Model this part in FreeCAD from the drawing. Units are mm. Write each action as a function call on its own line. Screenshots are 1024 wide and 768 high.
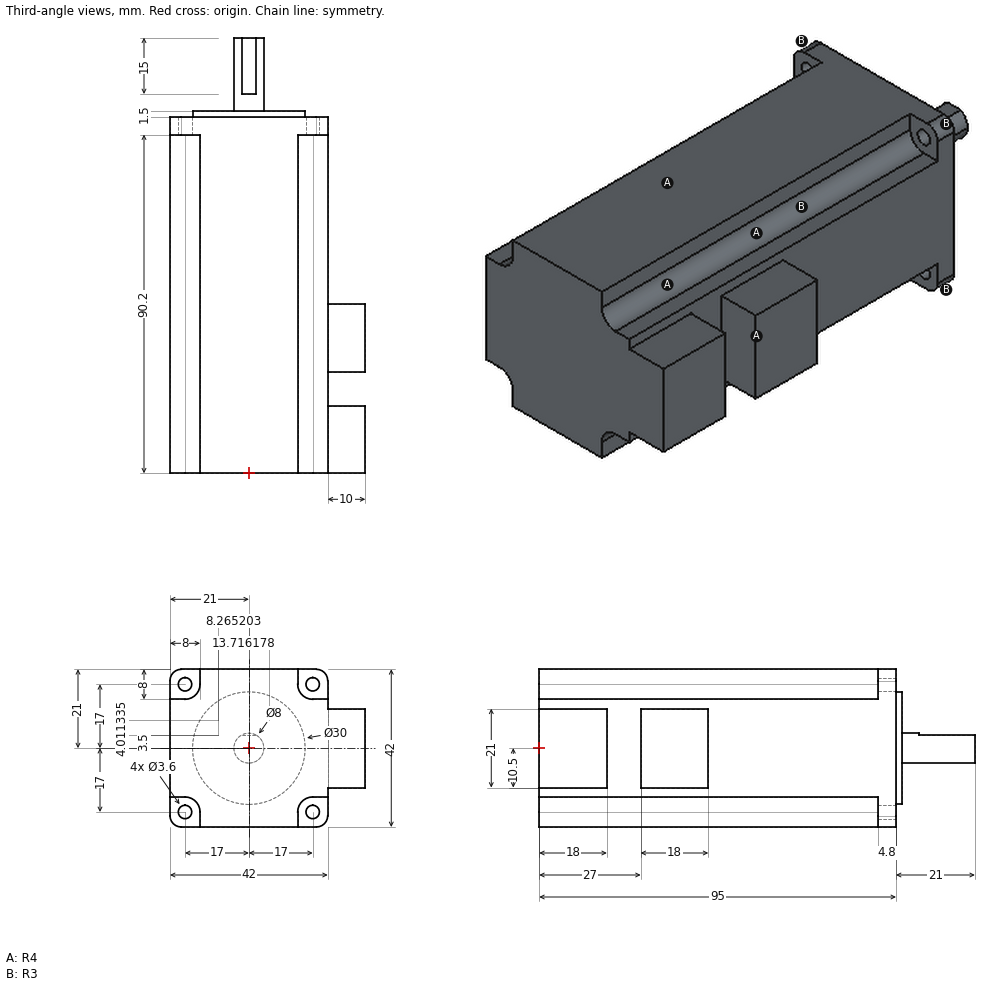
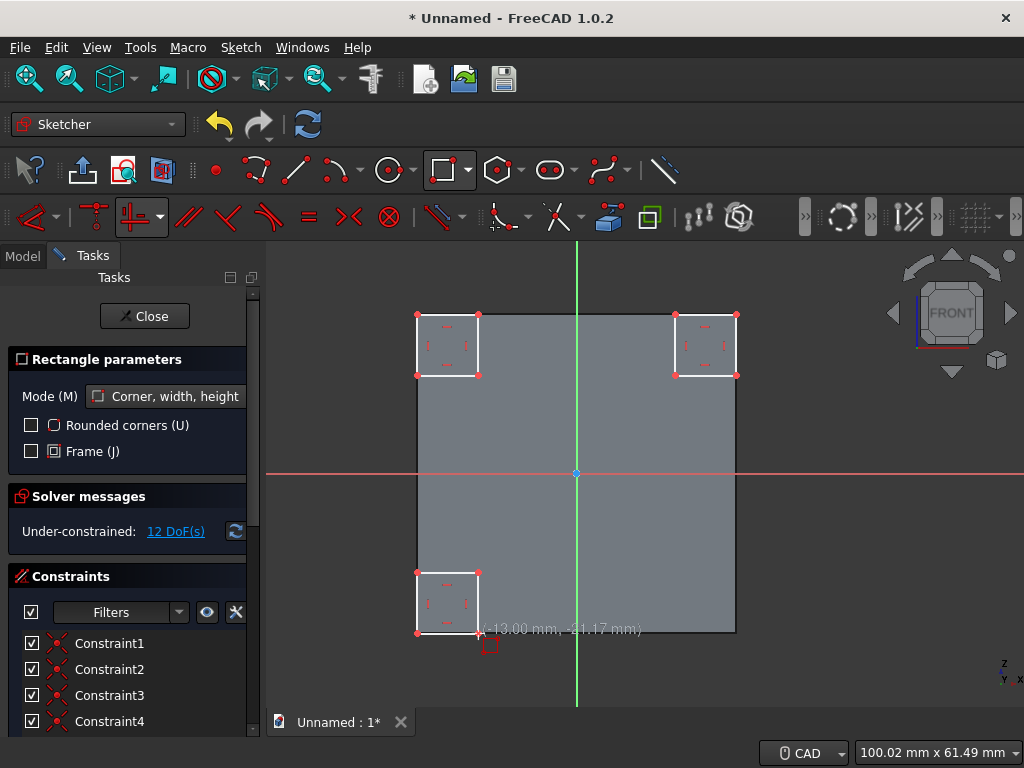
click(675, 572)
click(736, 633)
key(Escape)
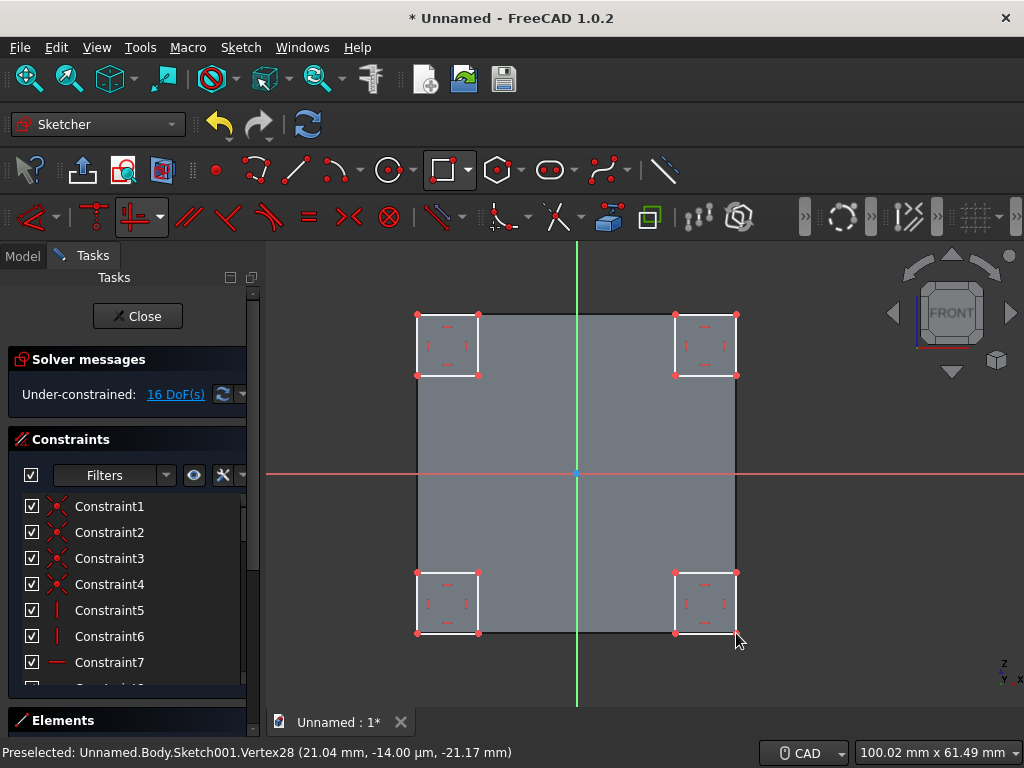
click(478, 315)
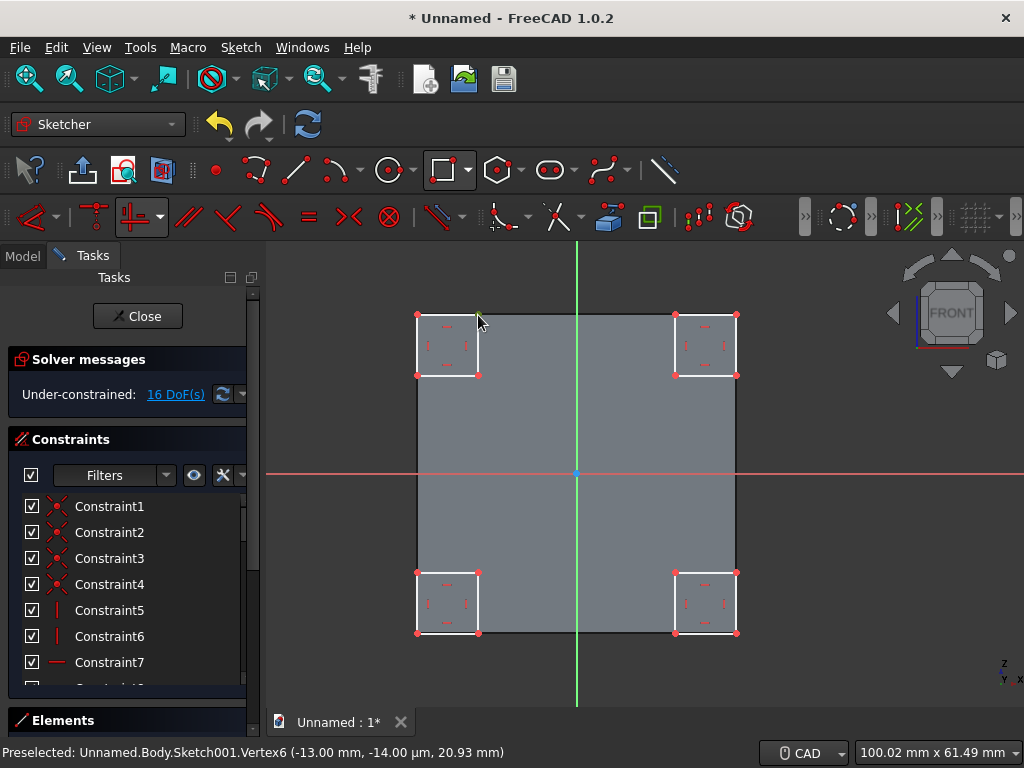
click(675, 315)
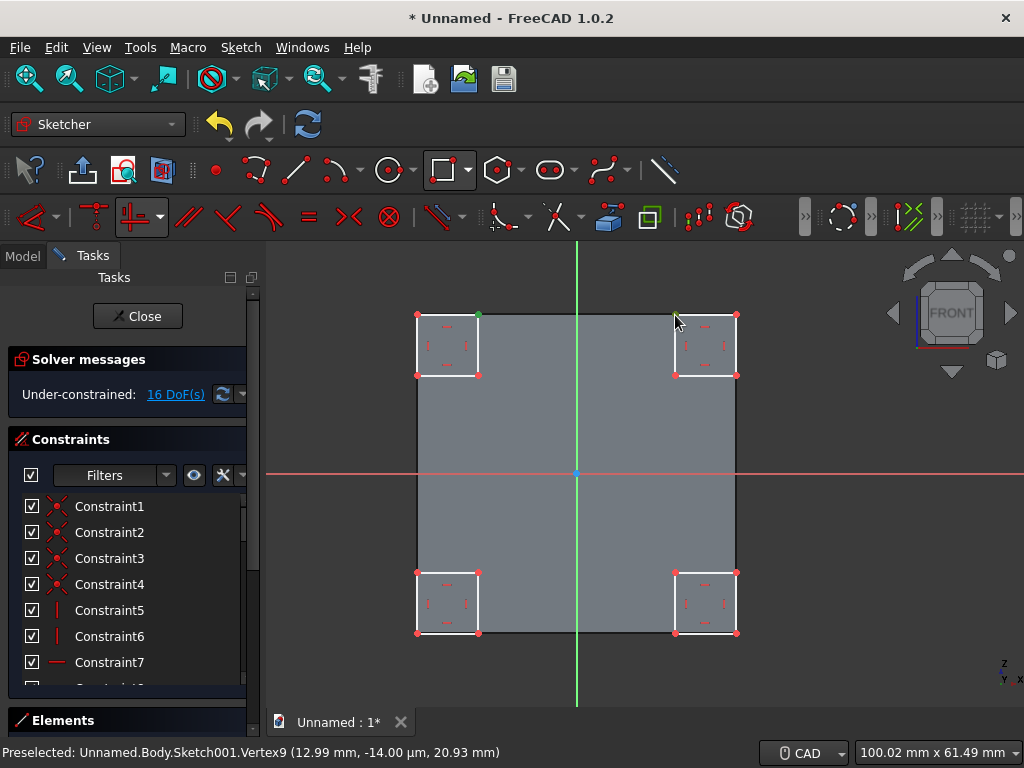
click(577, 650)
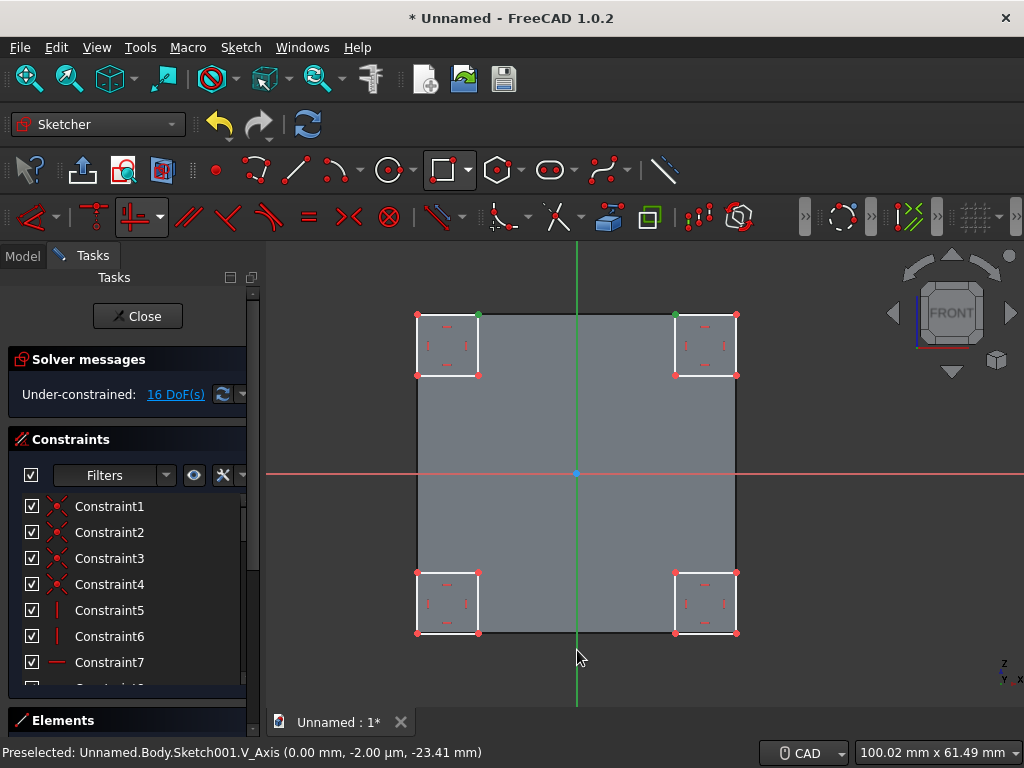
click(350, 218)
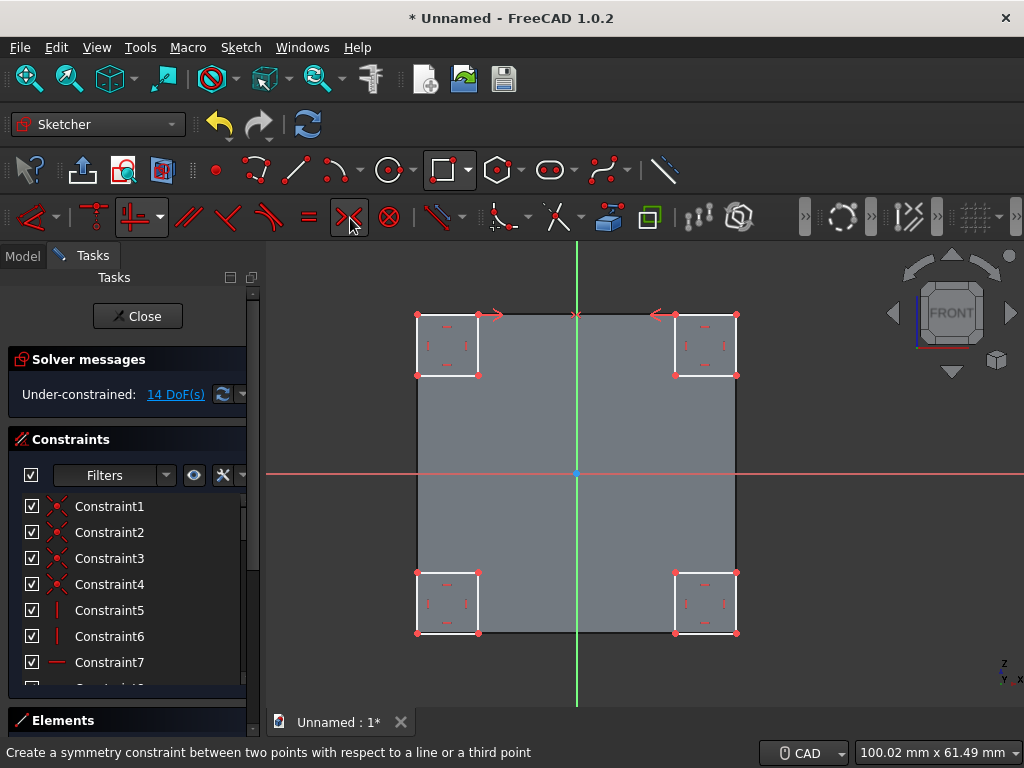
click(417, 376)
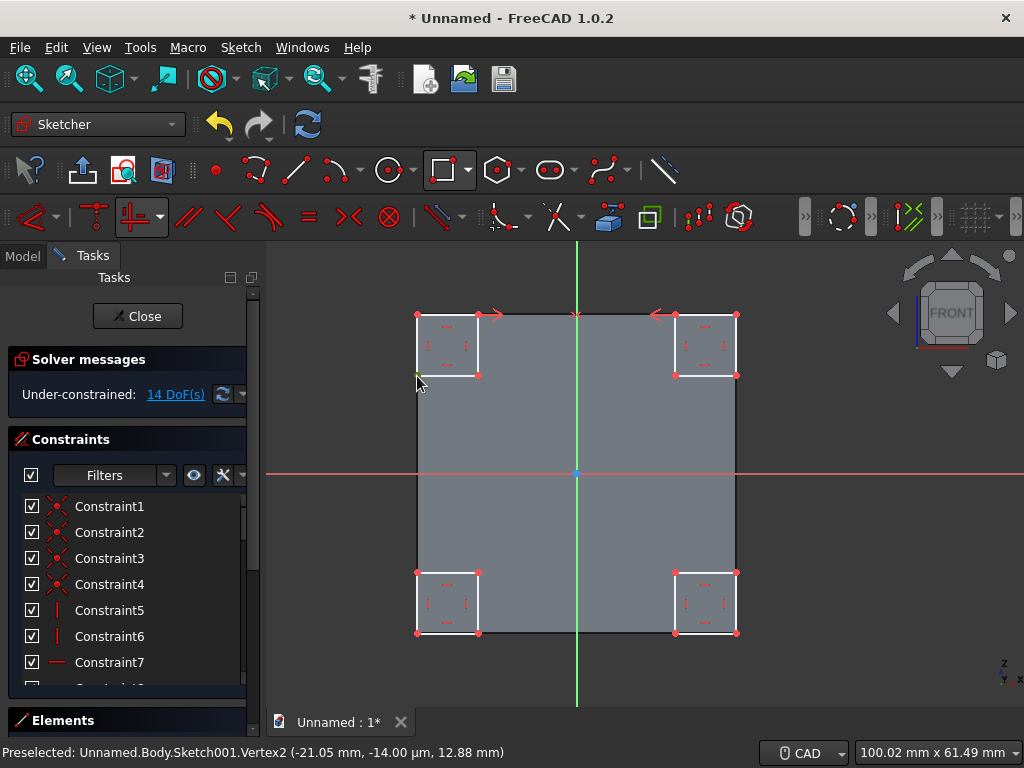
click(736, 376)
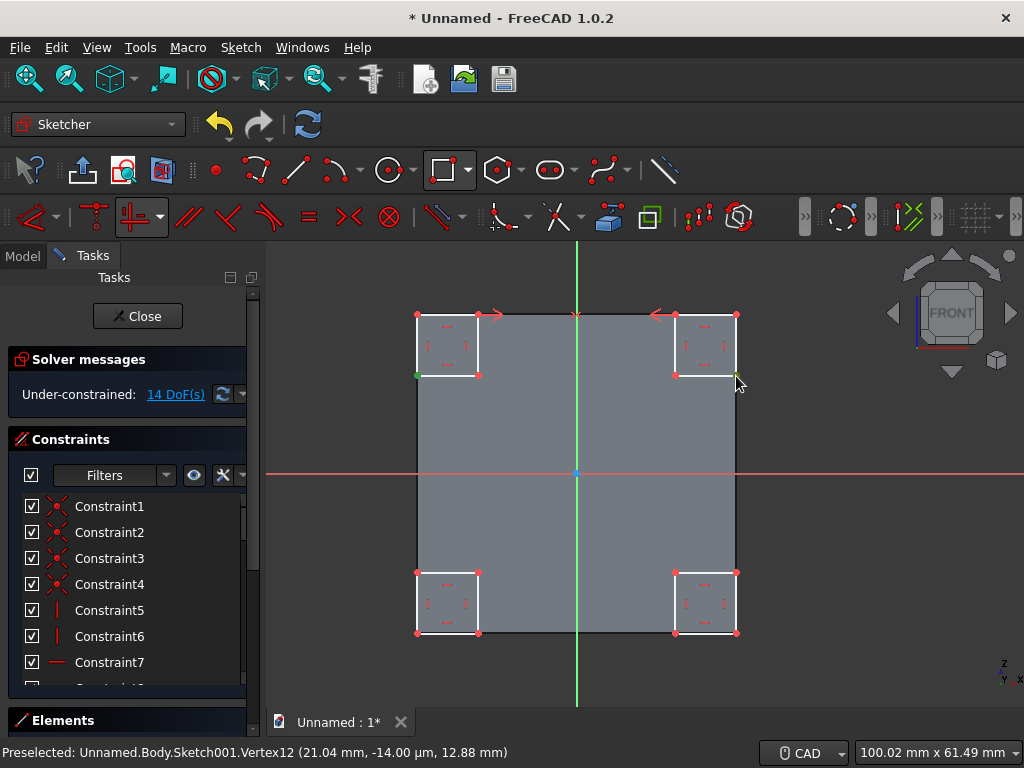
click(577, 650)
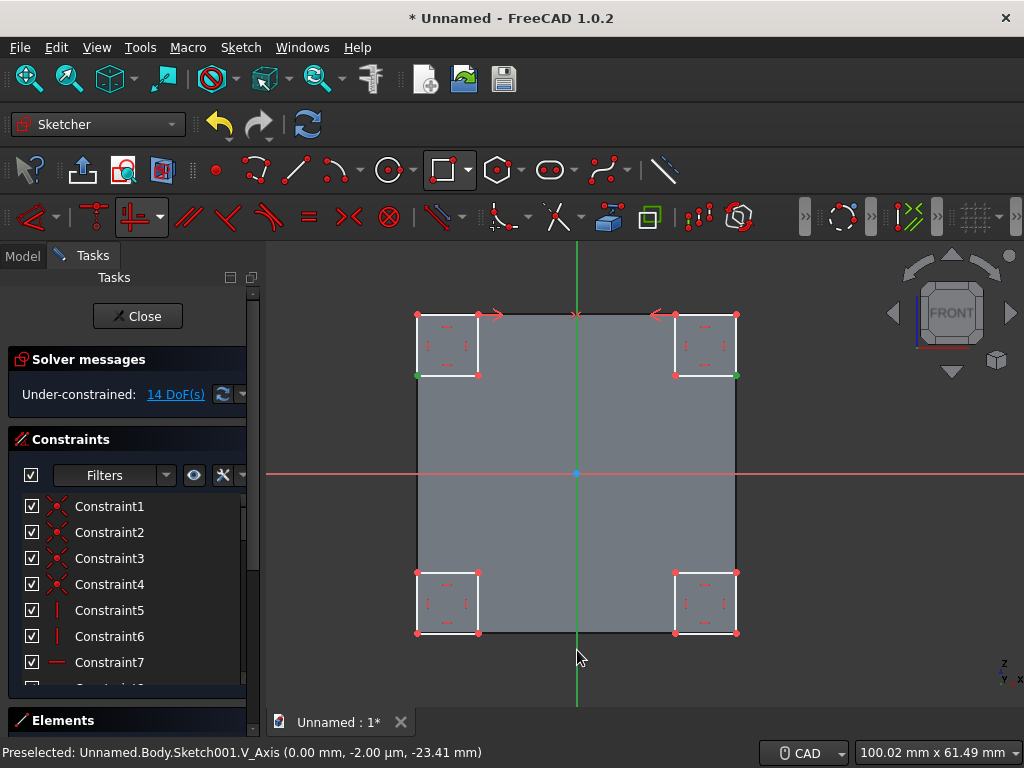
click(350, 218)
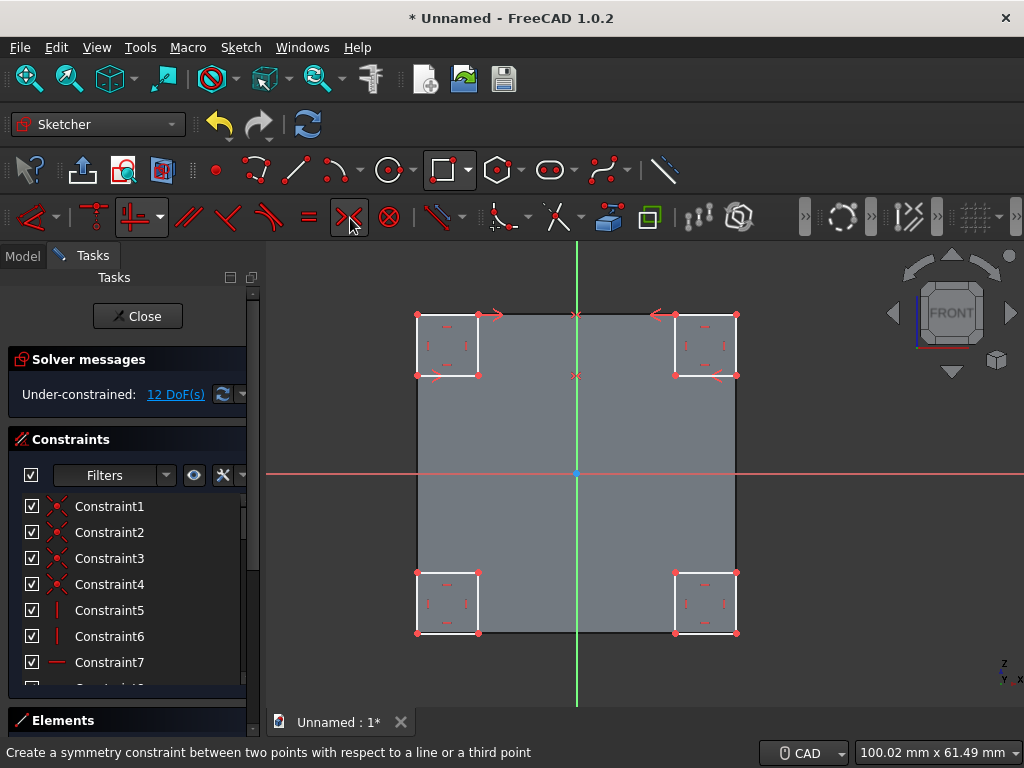
click(417, 376)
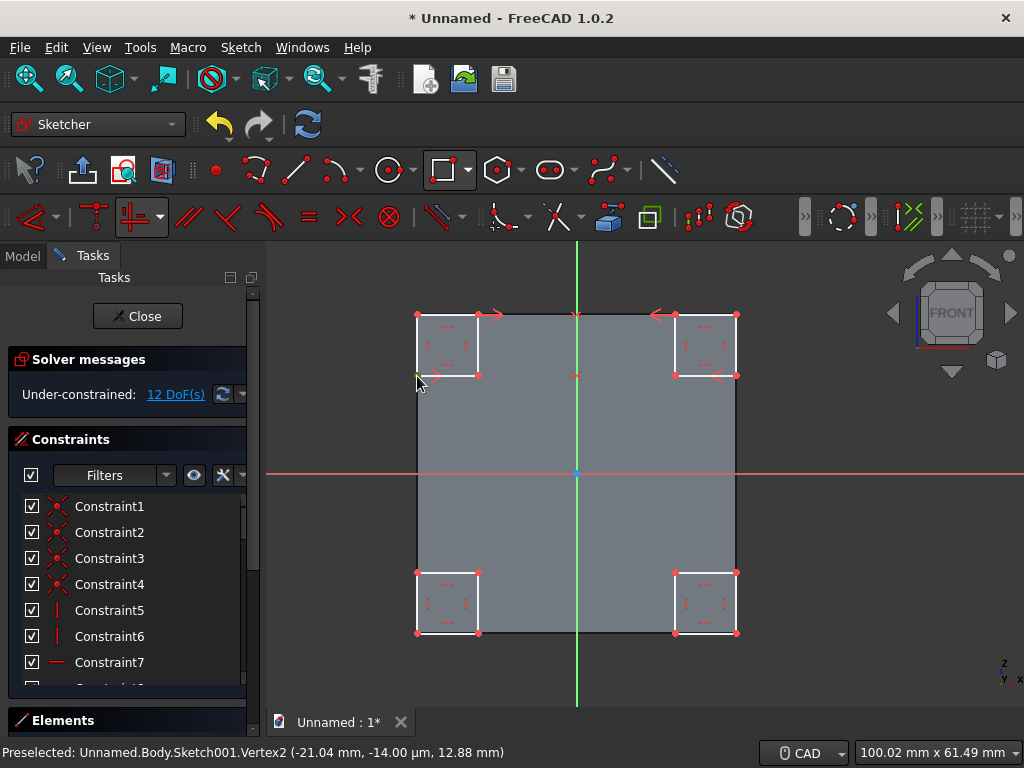
click(417, 573)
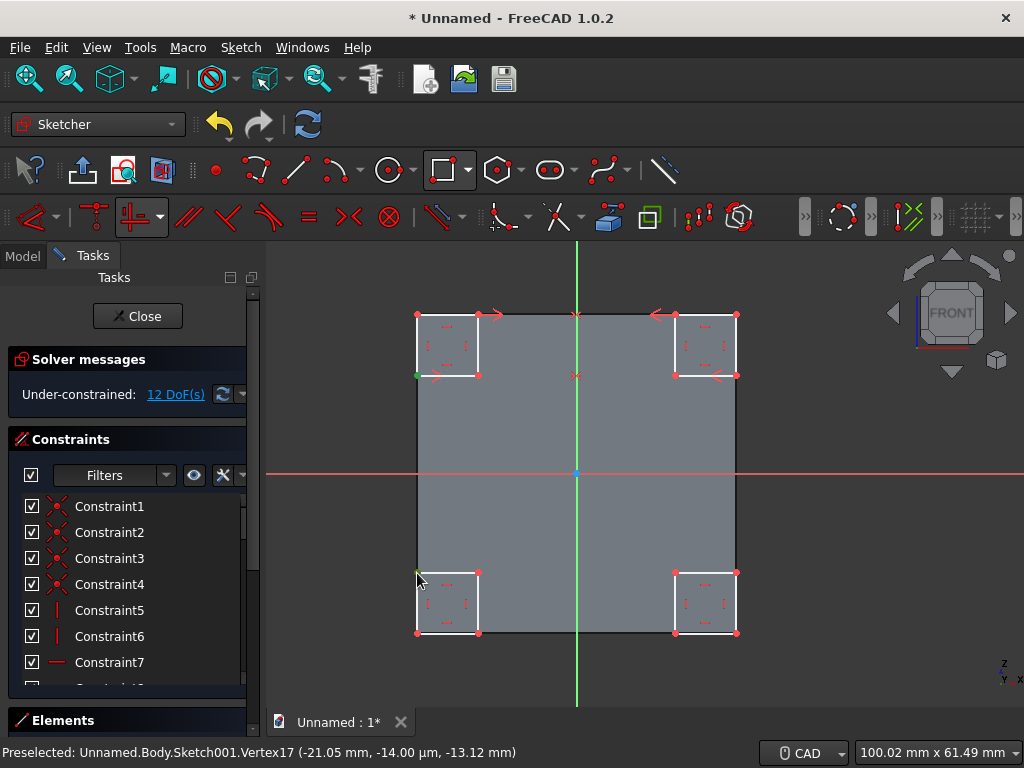
click(334, 474)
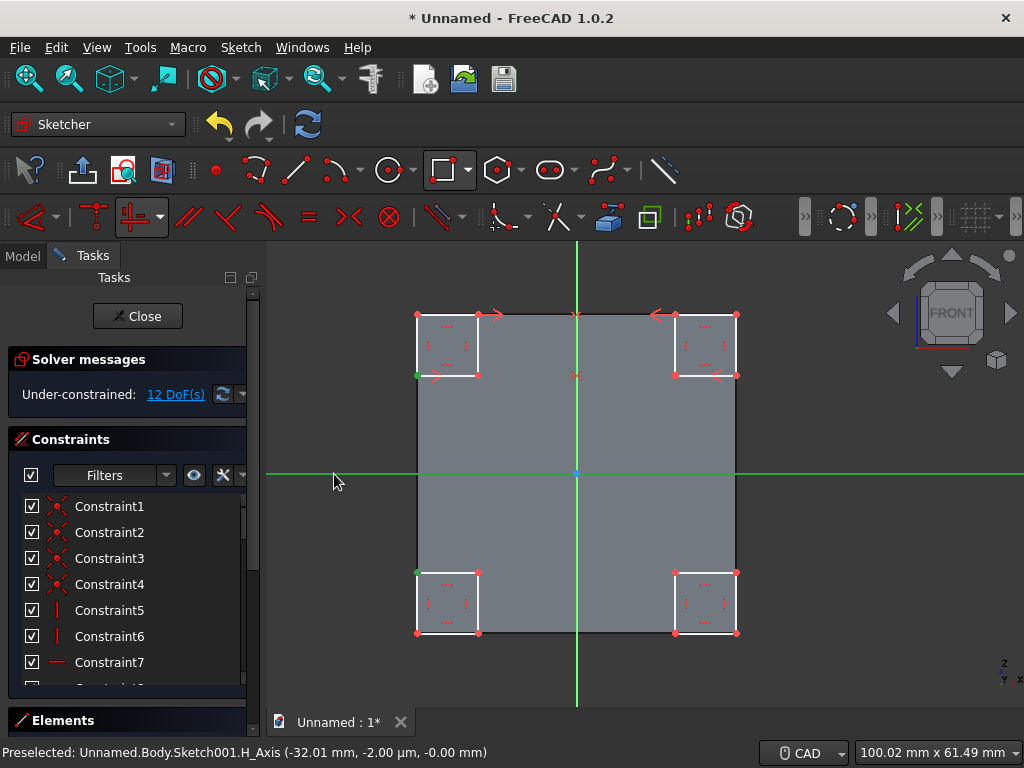
click(350, 218)